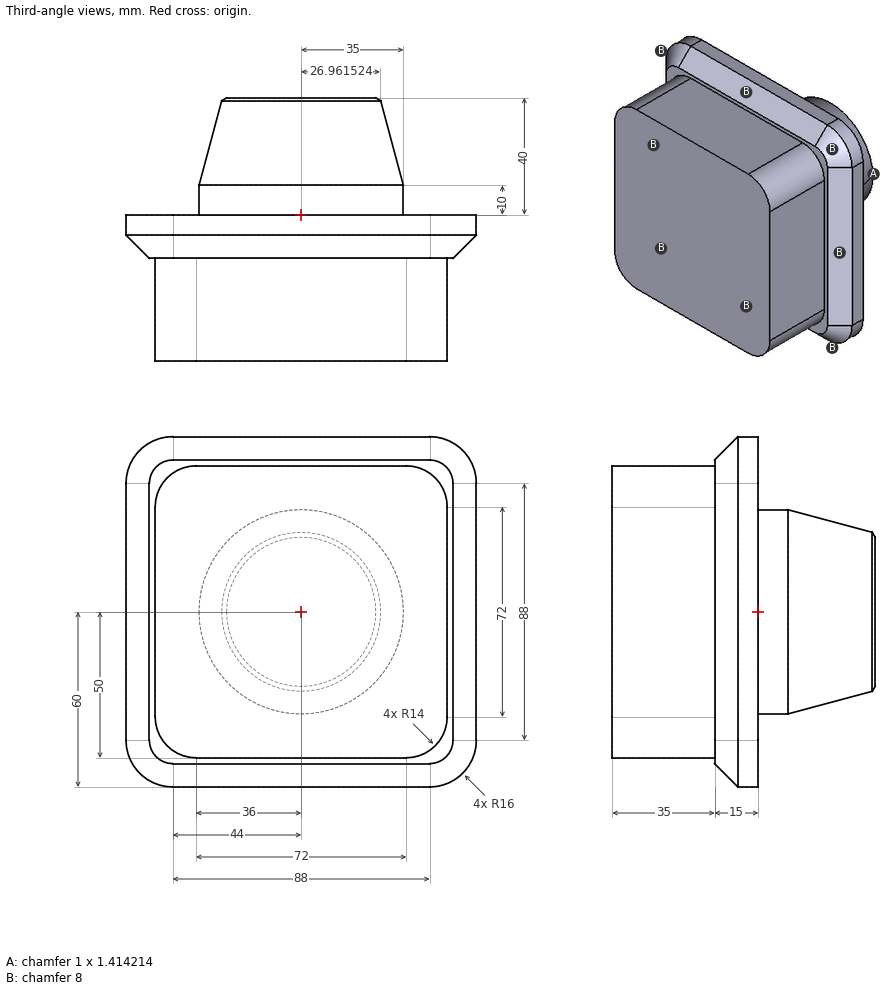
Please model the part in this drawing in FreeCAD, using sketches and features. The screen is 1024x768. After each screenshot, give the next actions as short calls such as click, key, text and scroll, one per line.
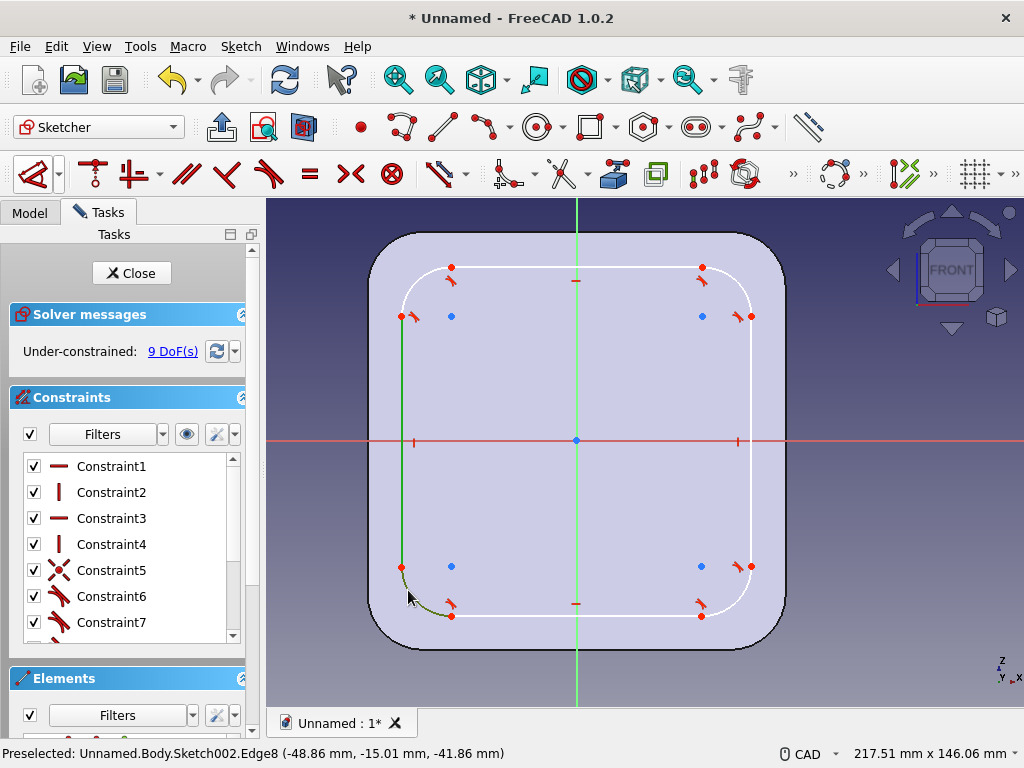
click(269, 174)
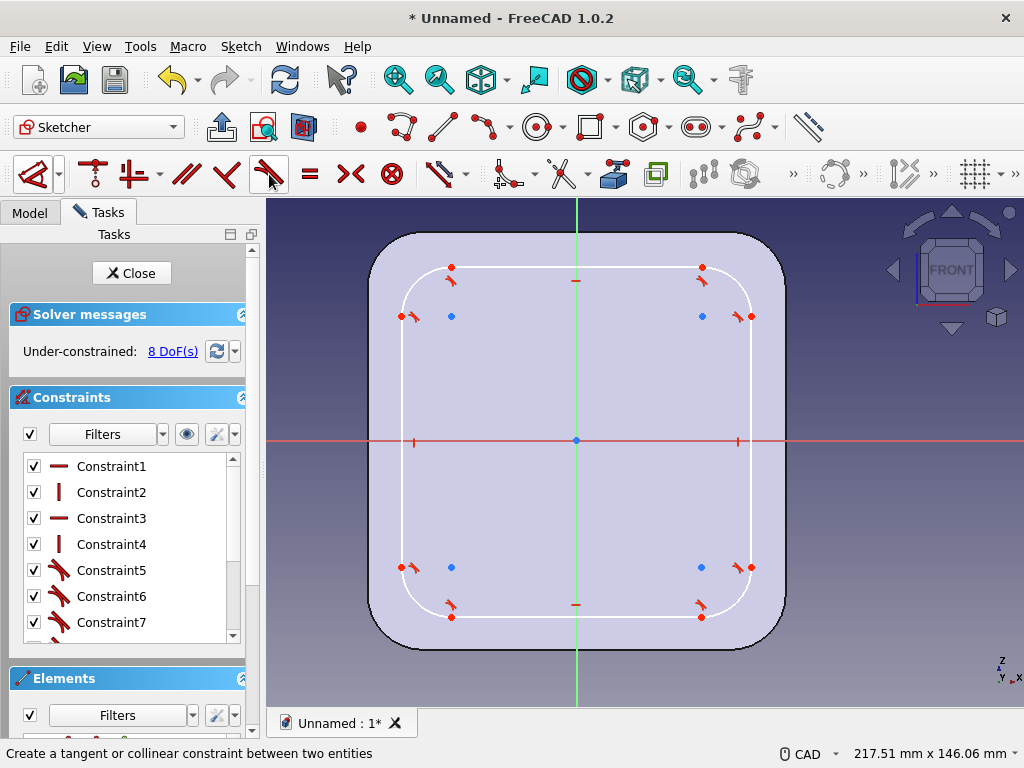
click(724, 612)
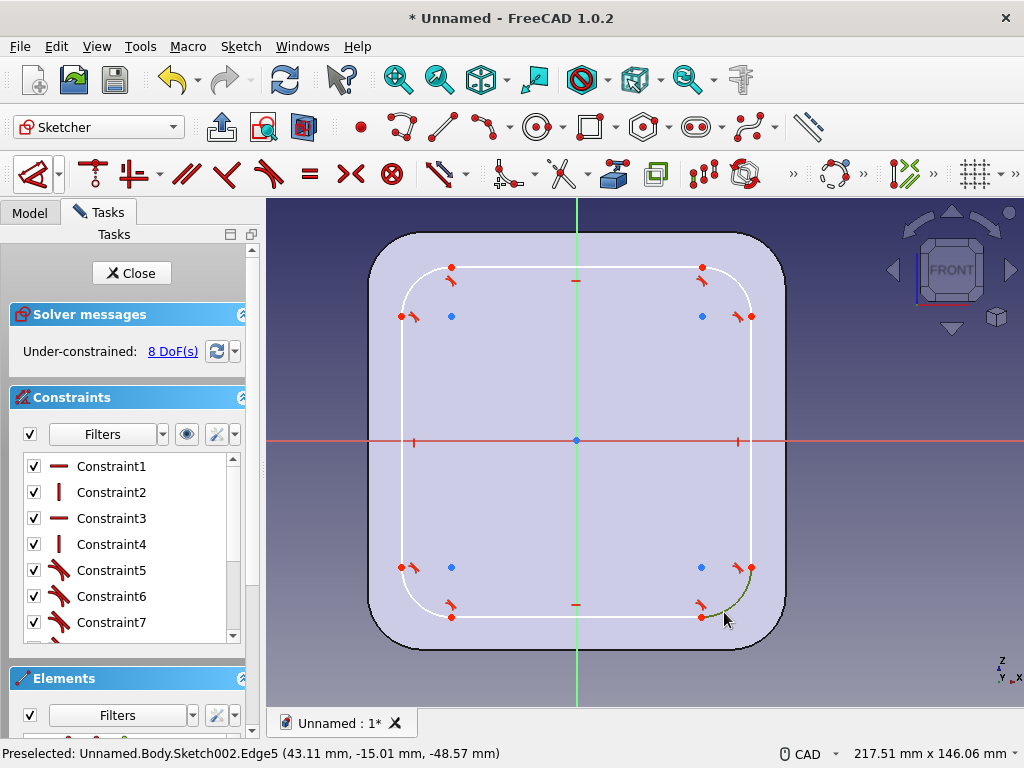
click(746, 294)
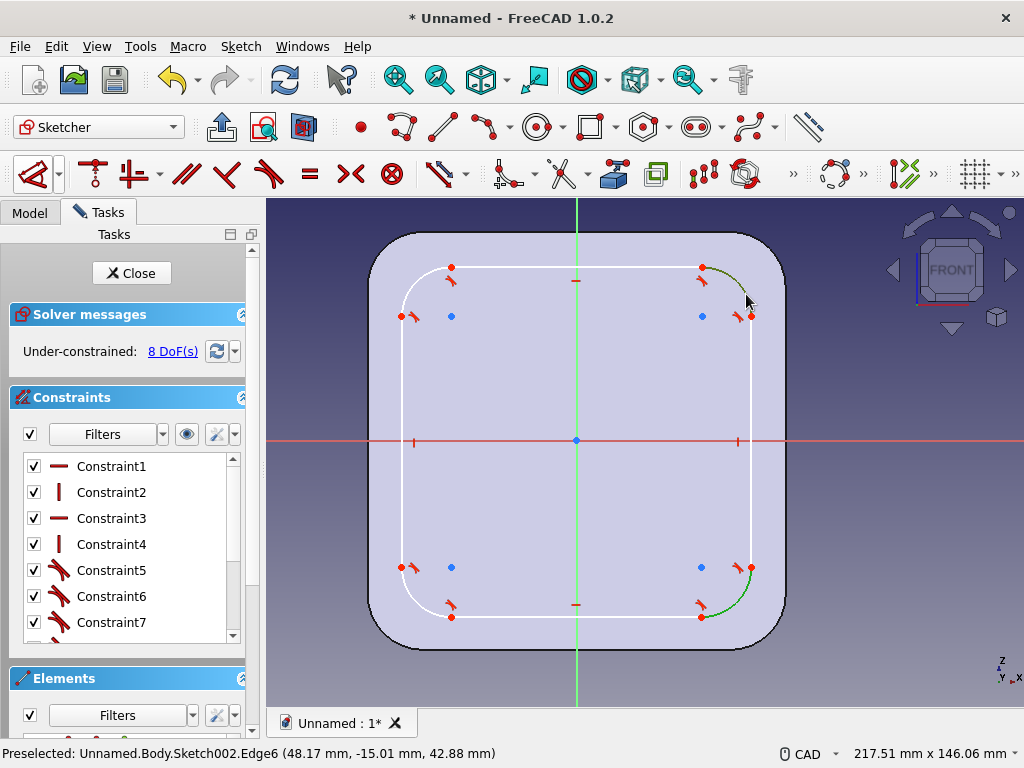
click(429, 273)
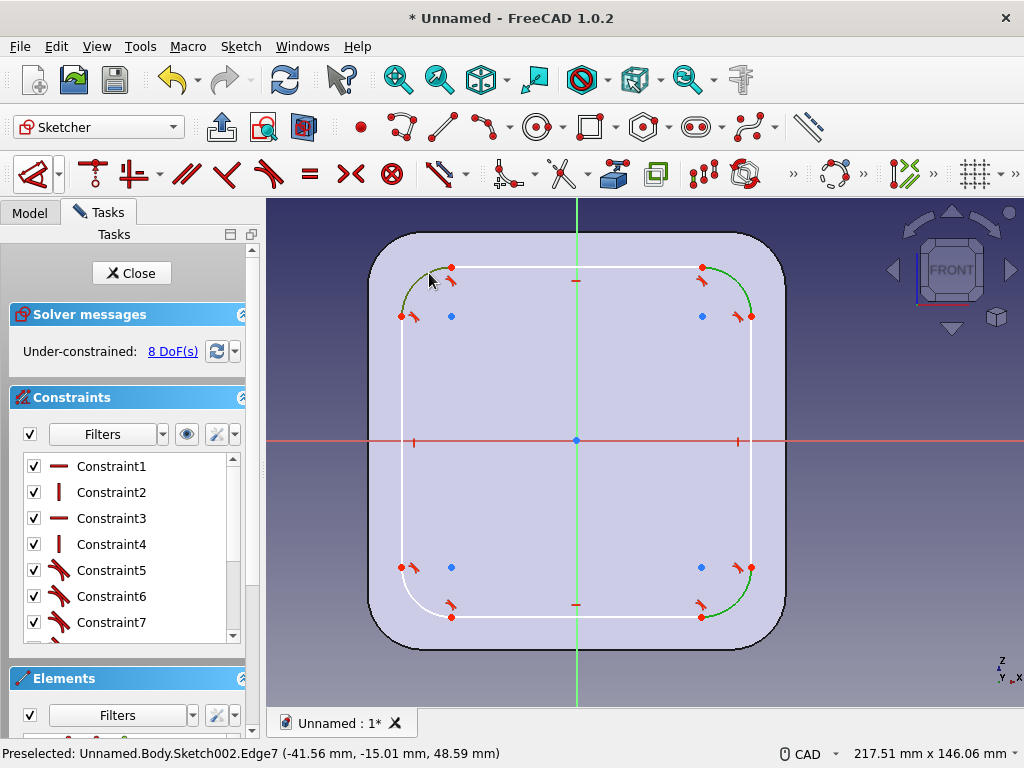
click(407, 590)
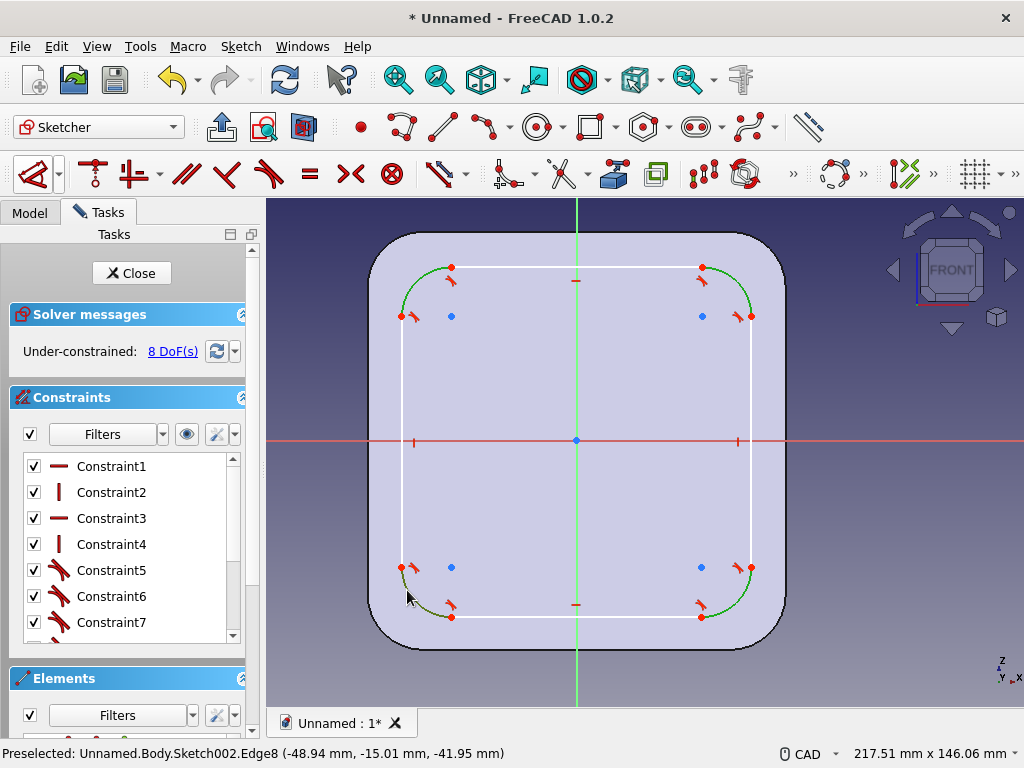
key(e)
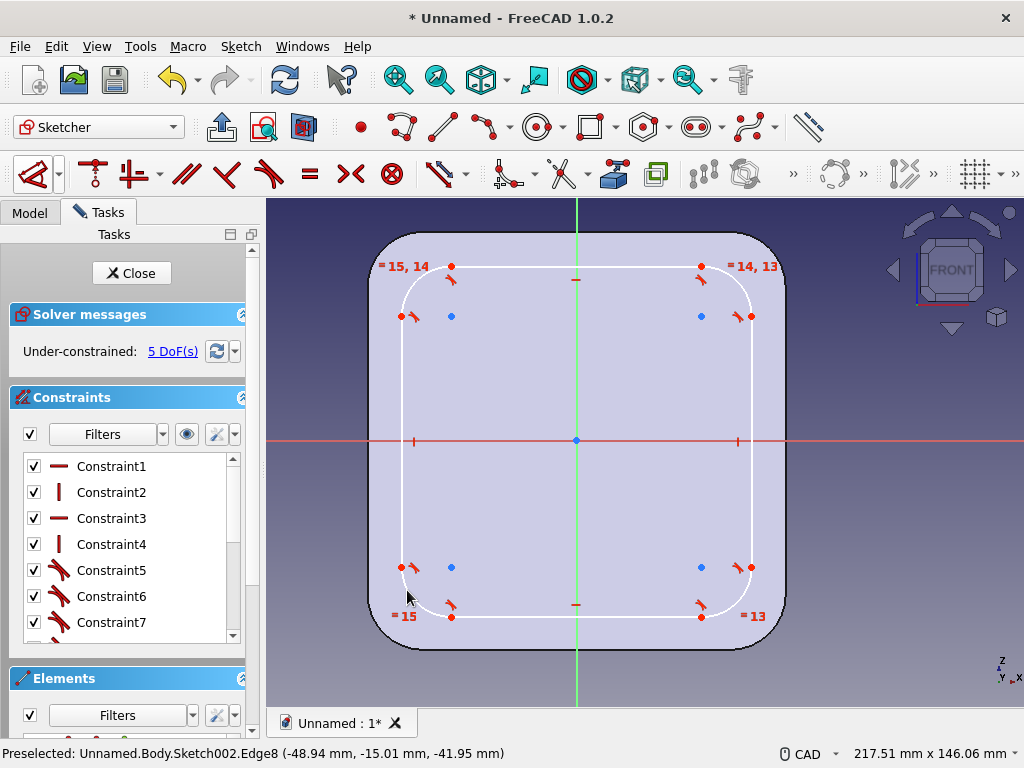
key(d)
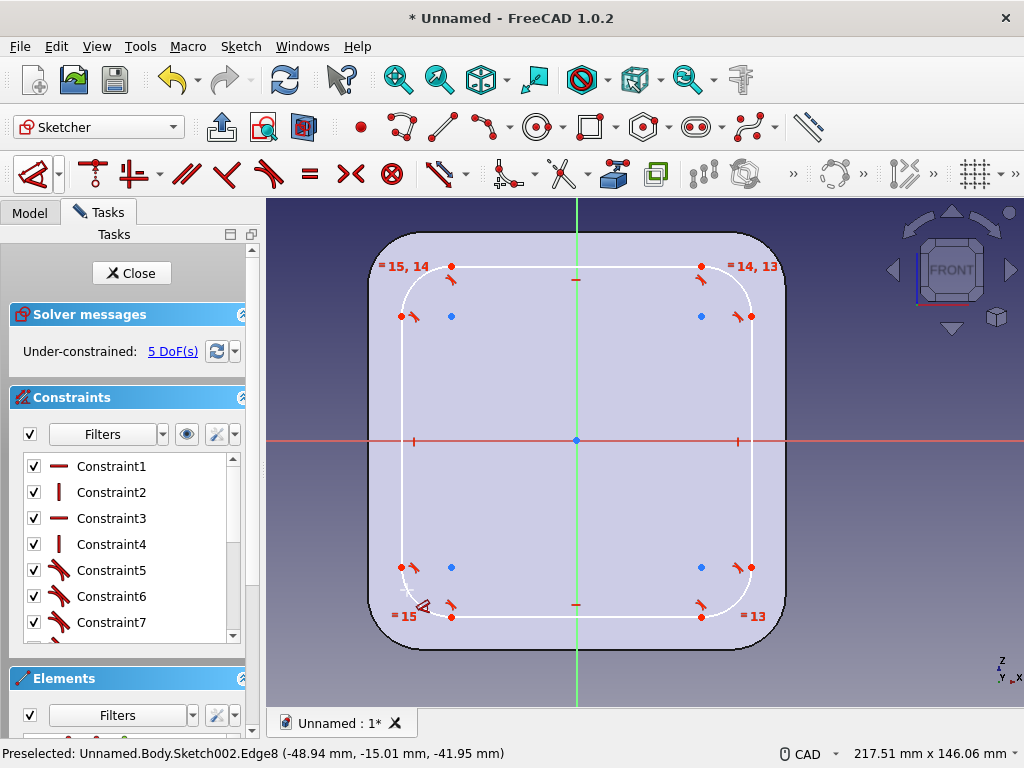
click(724, 612)
click(738, 641)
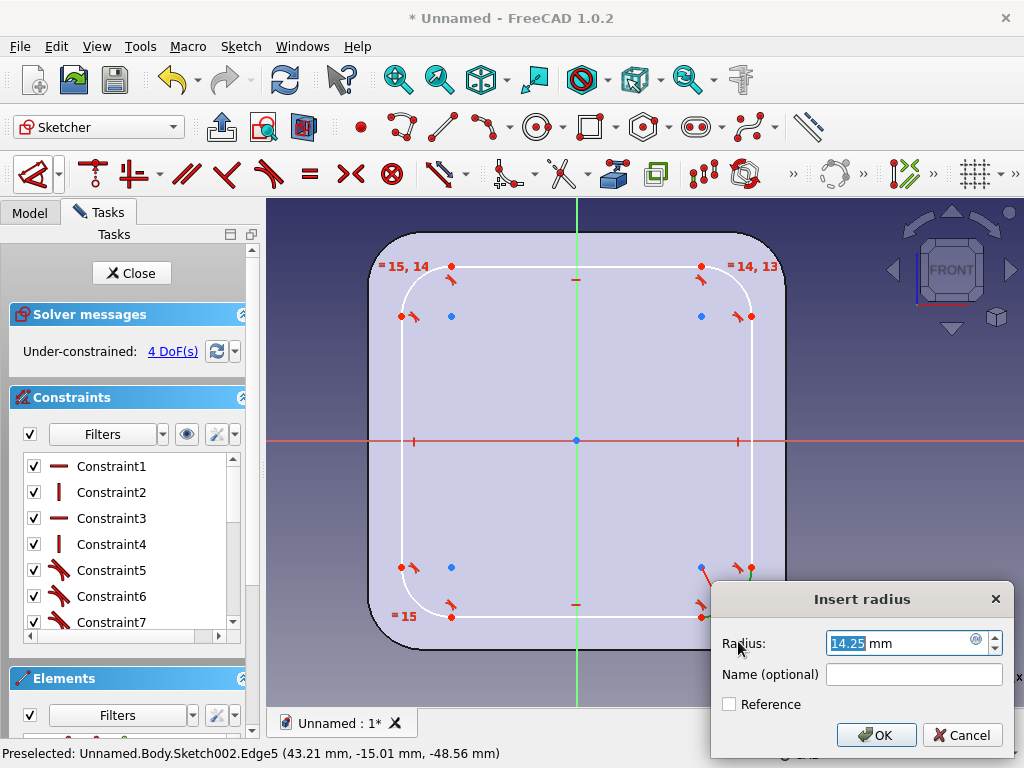
text(14)
key(Return)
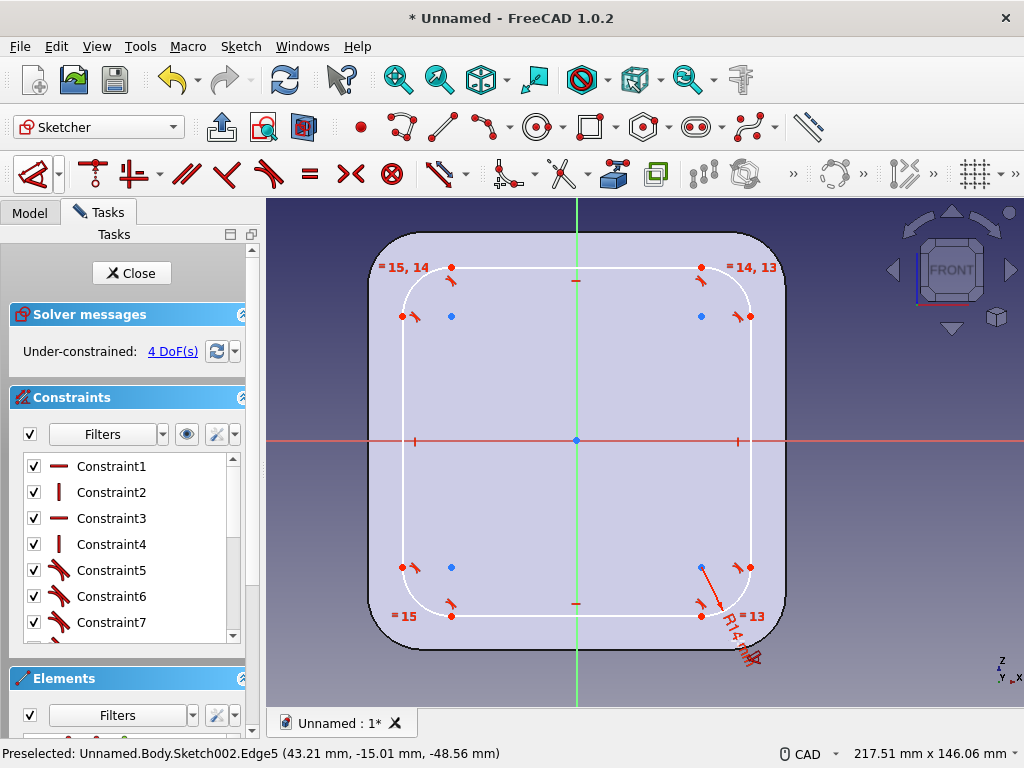
click(527, 616)
click(519, 650)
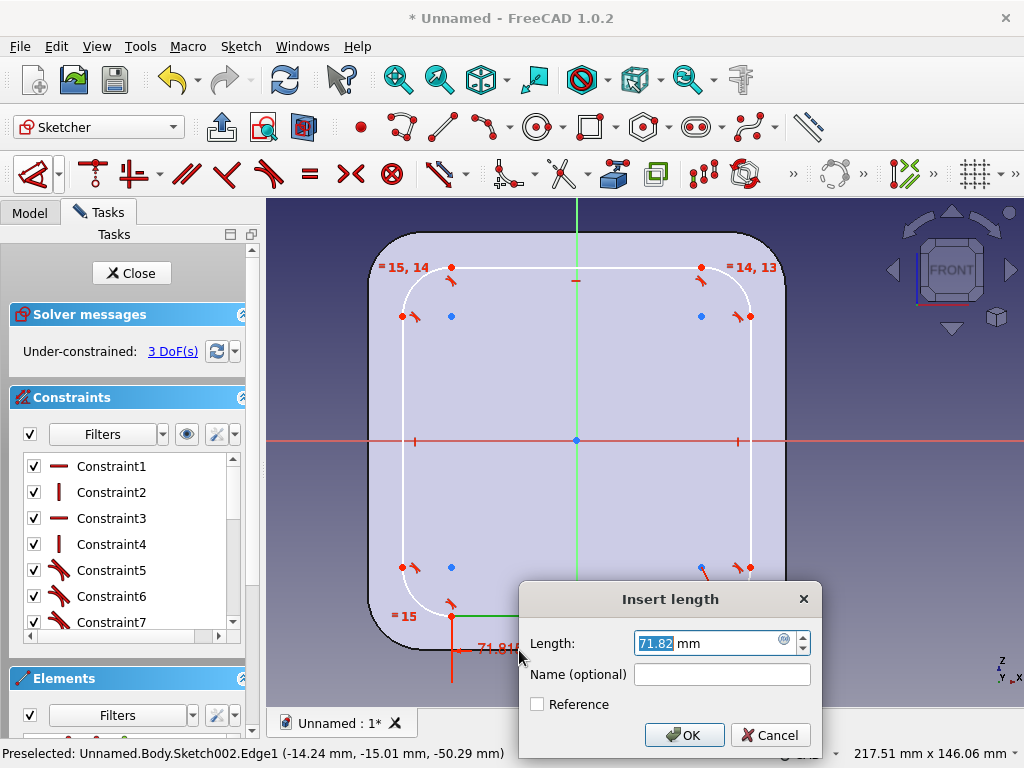
text(72)
key(Return)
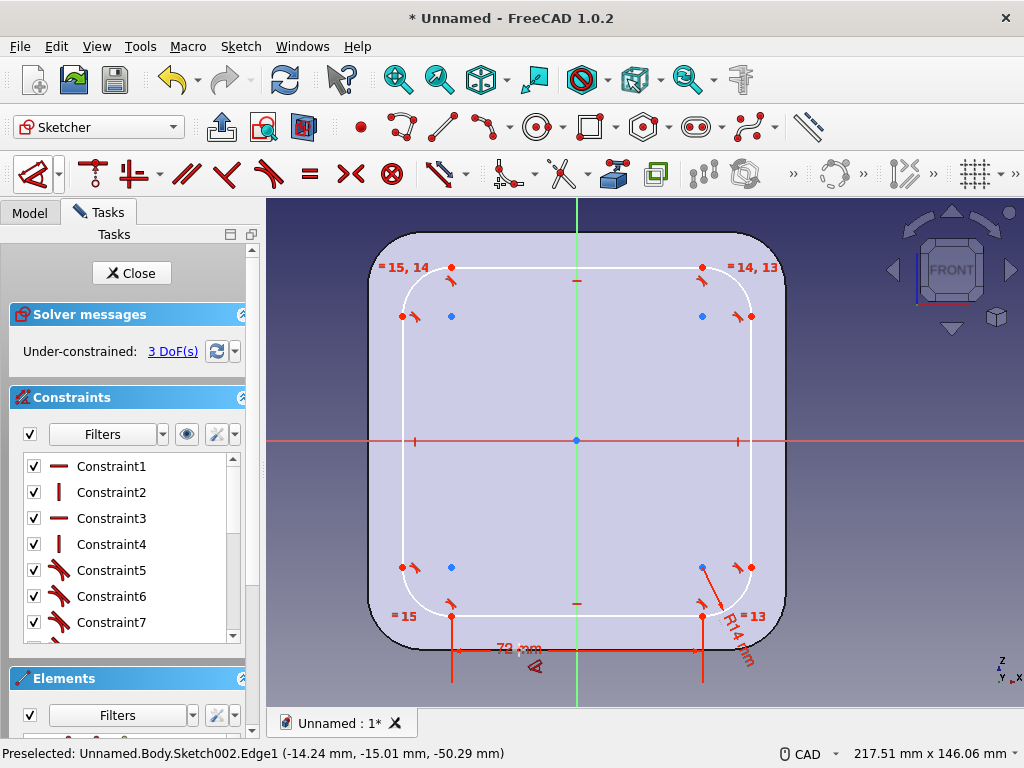
click(751, 492)
click(785, 384)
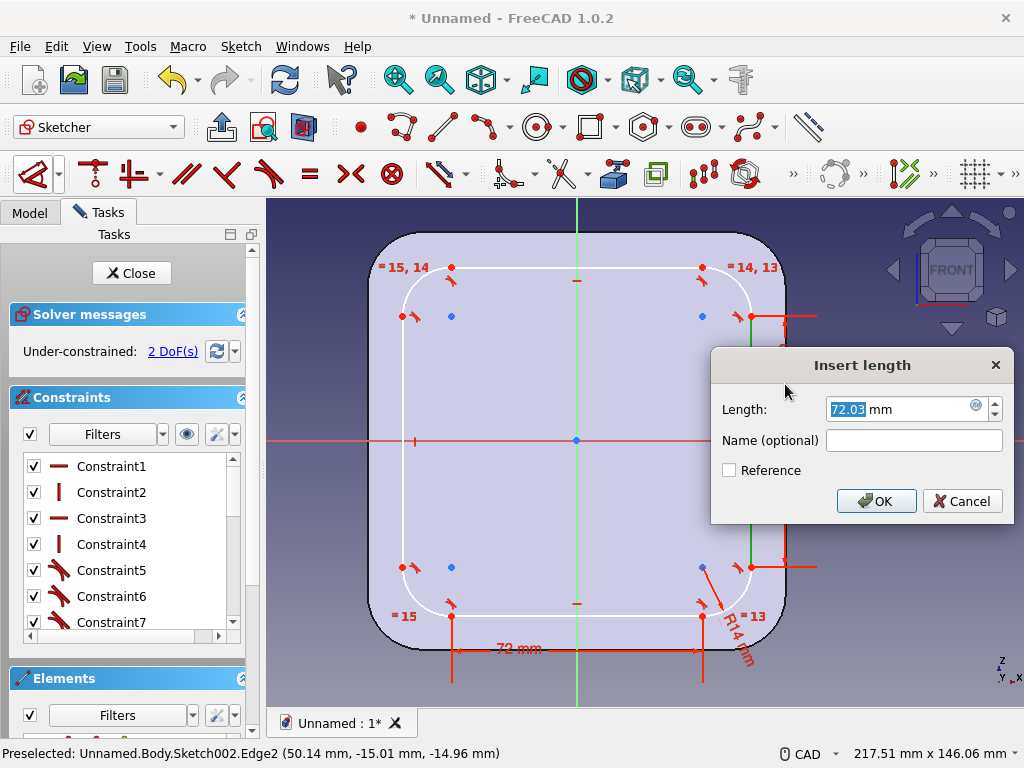
text(72)
key(Return)